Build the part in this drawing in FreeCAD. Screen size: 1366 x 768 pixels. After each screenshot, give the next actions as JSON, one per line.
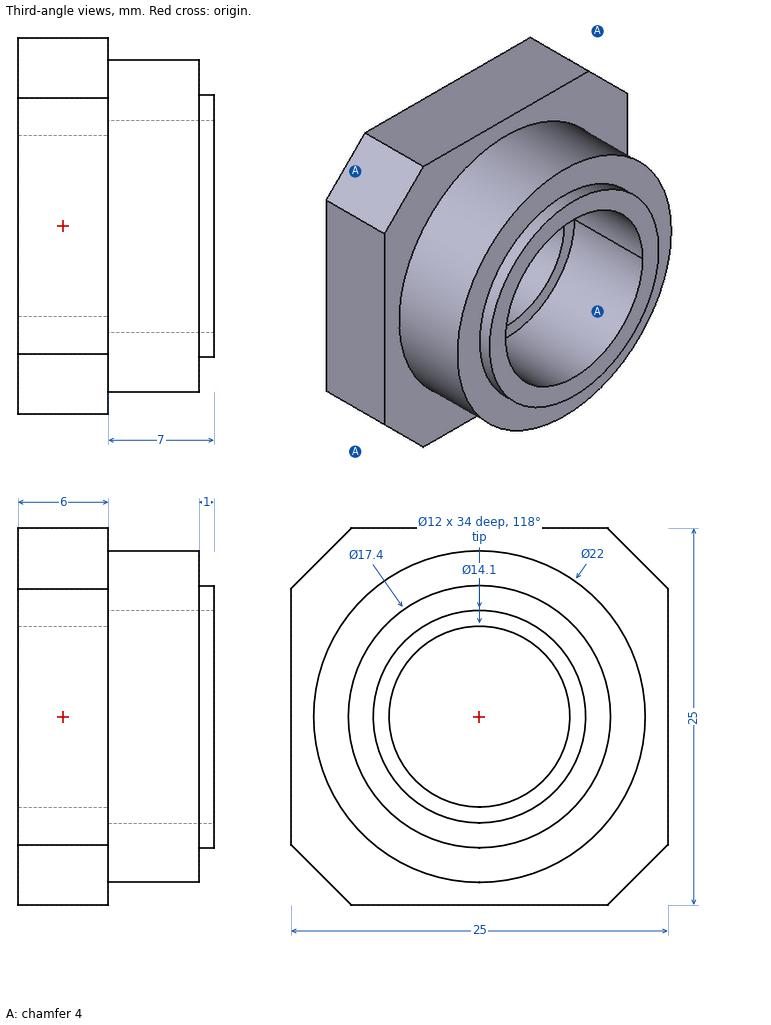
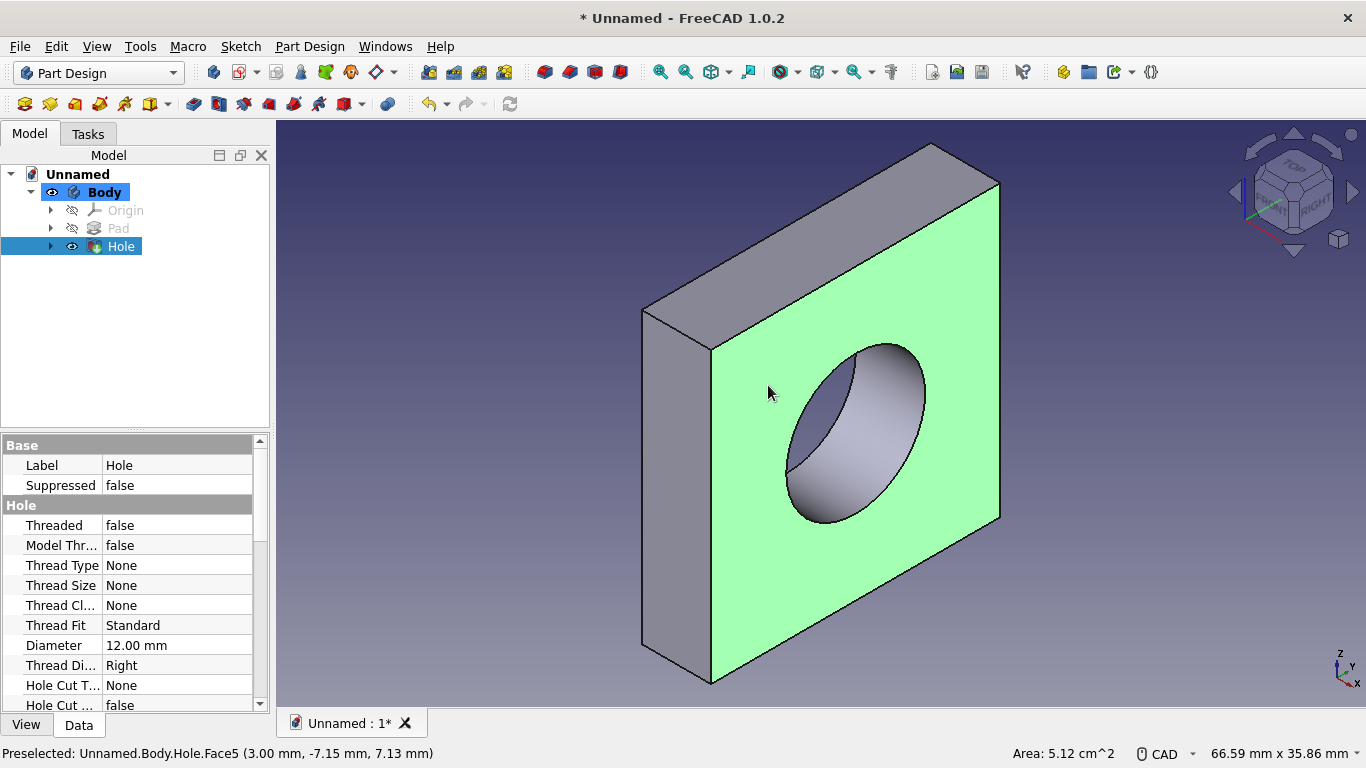
{"action": "left_click", "coordinate": [238, 72]}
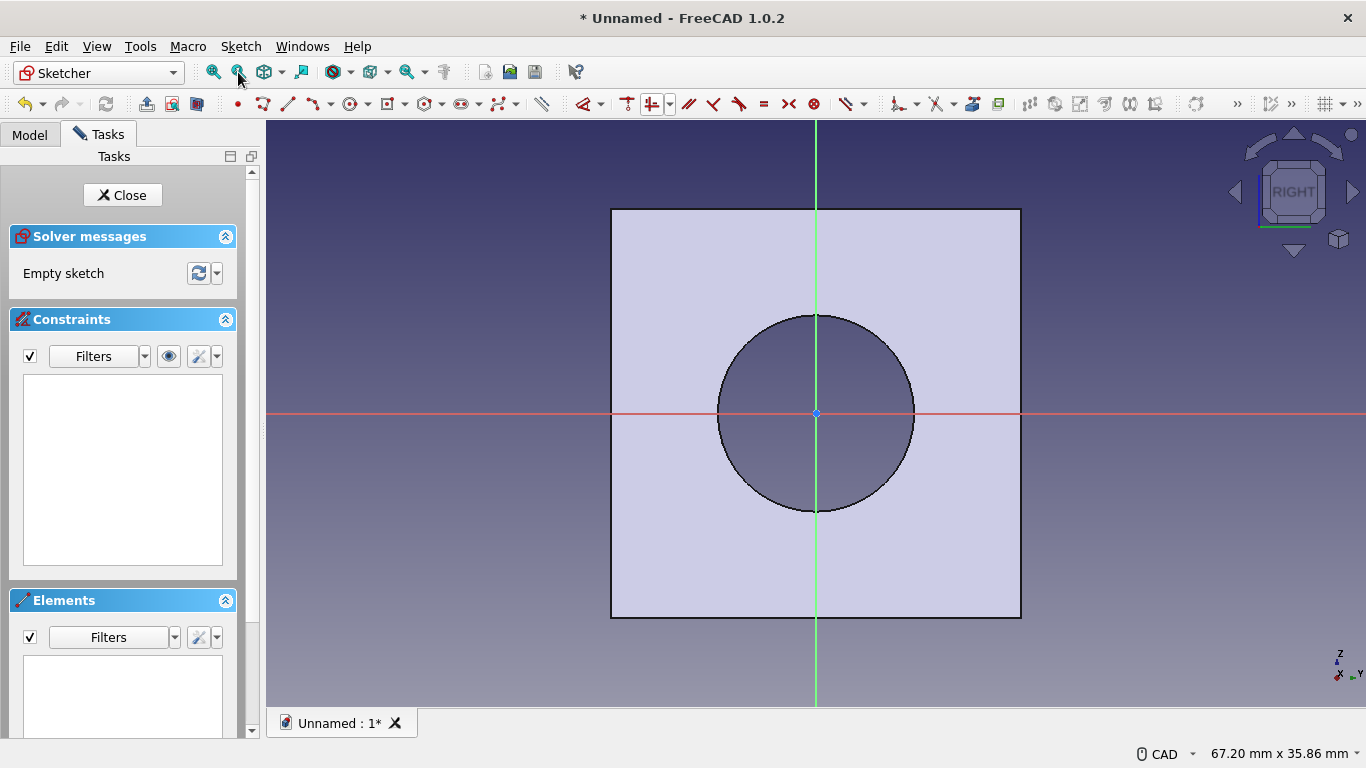
{"action": "left_click", "coordinate": [350, 104]}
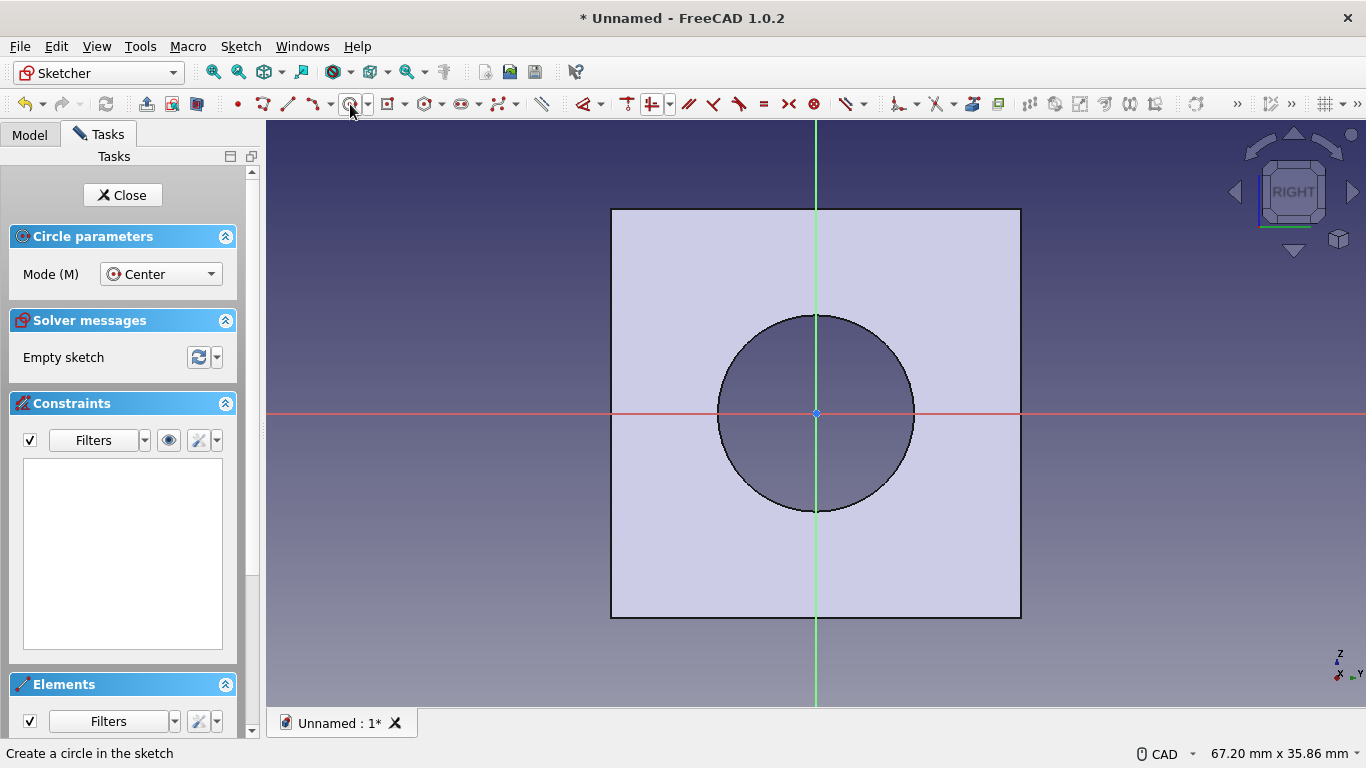
{"action": "left_click", "coordinate": [816, 414]}
{"action": "mouse_move", "coordinate": [943, 286]}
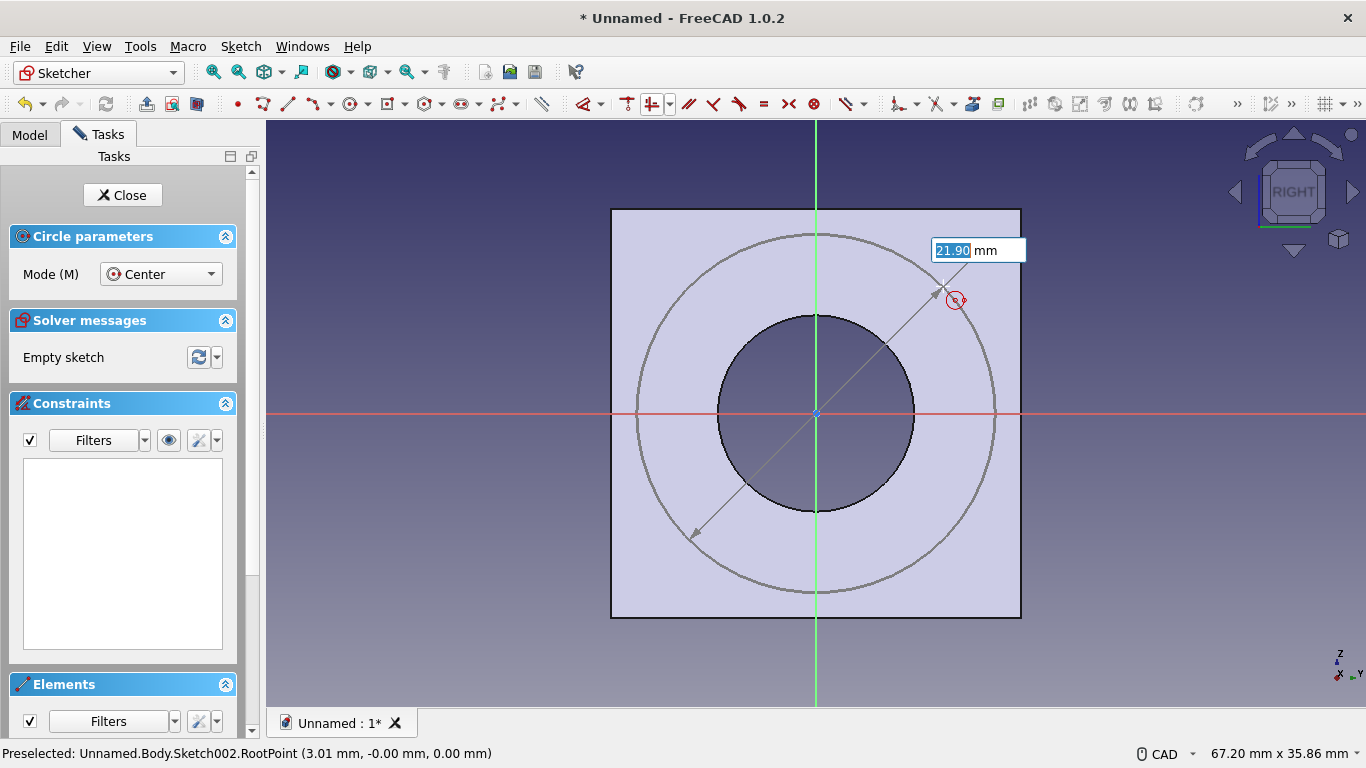
{"action": "type", "text": "22"}
{"action": "key", "text": "Return"}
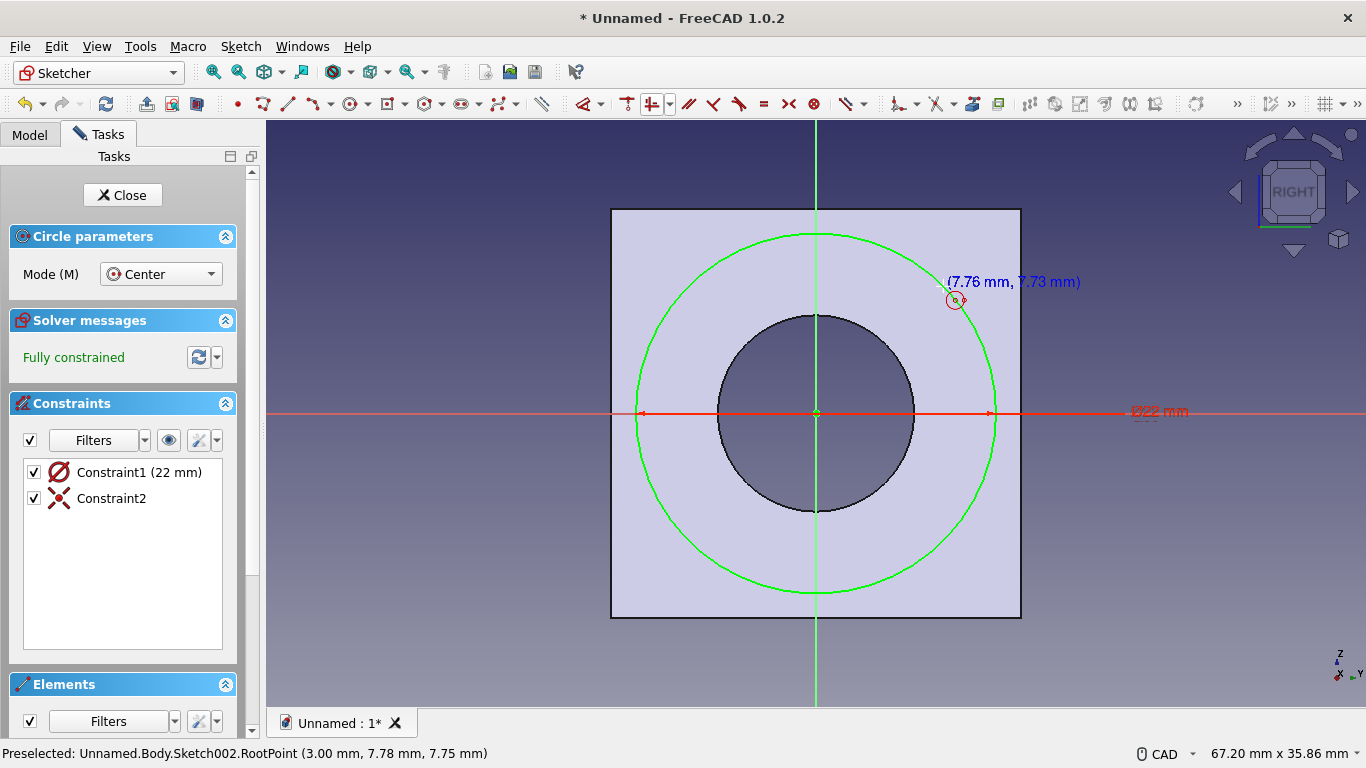
{"action": "left_click", "coordinate": [816, 414]}
{"action": "mouse_move", "coordinate": [898, 332]}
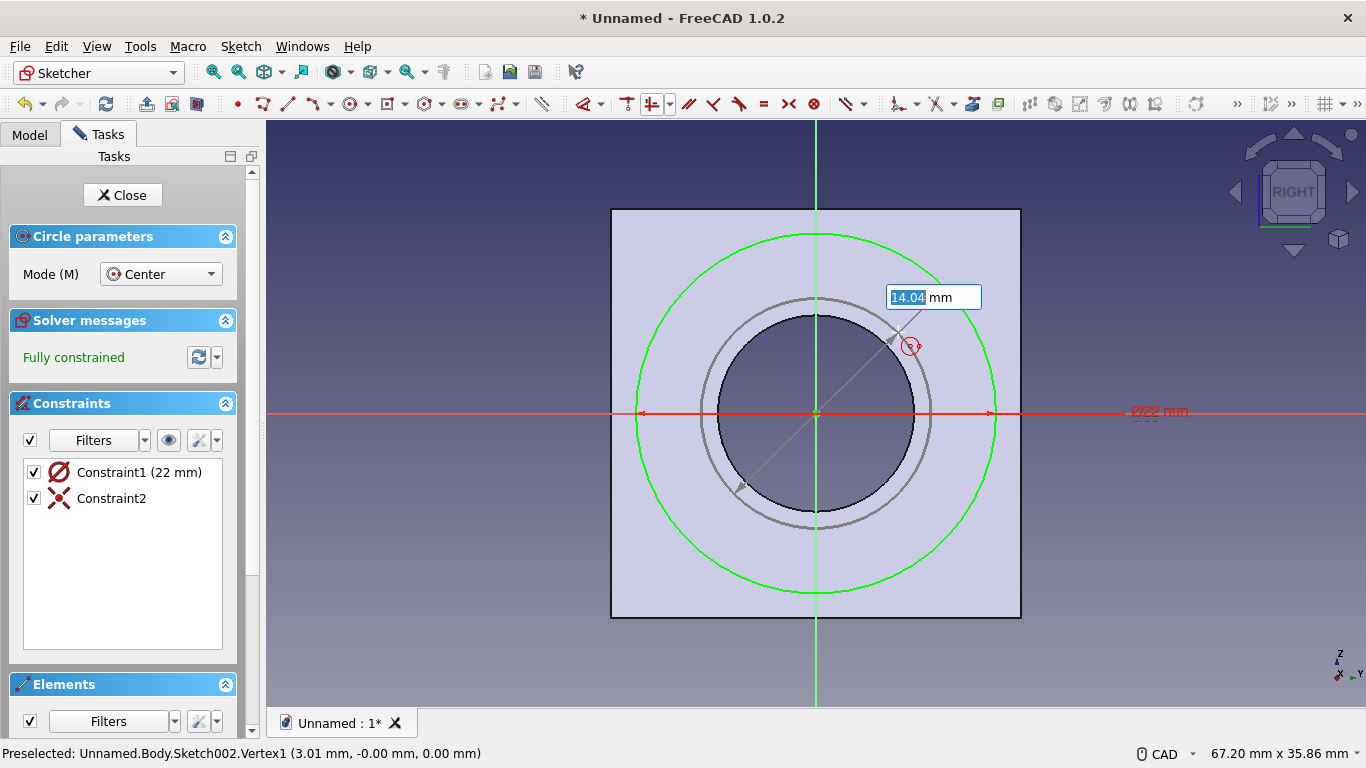
{"action": "type", "text": "14.1"}
{"action": "key", "text": "Return"}
{"action": "key", "text": "Escape"}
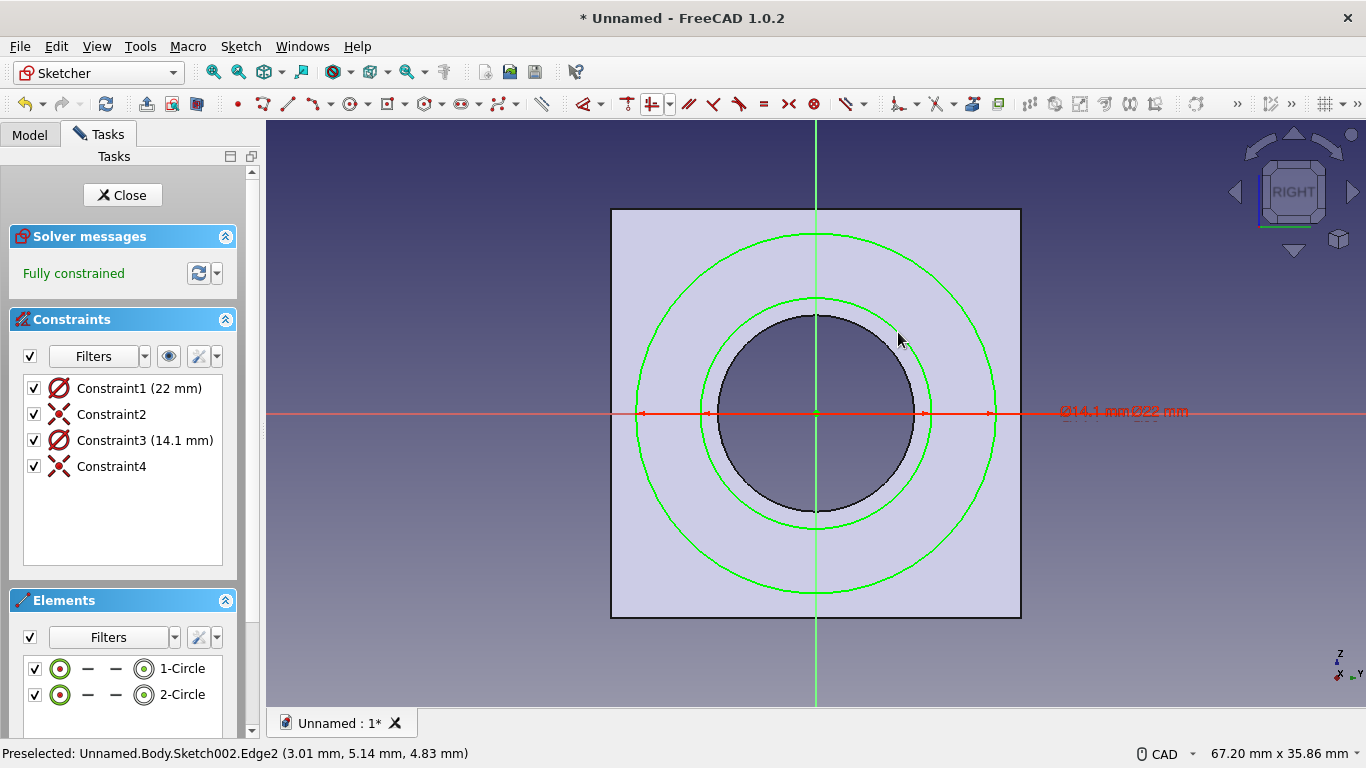
{"action": "left_click", "coordinate": [123, 195]}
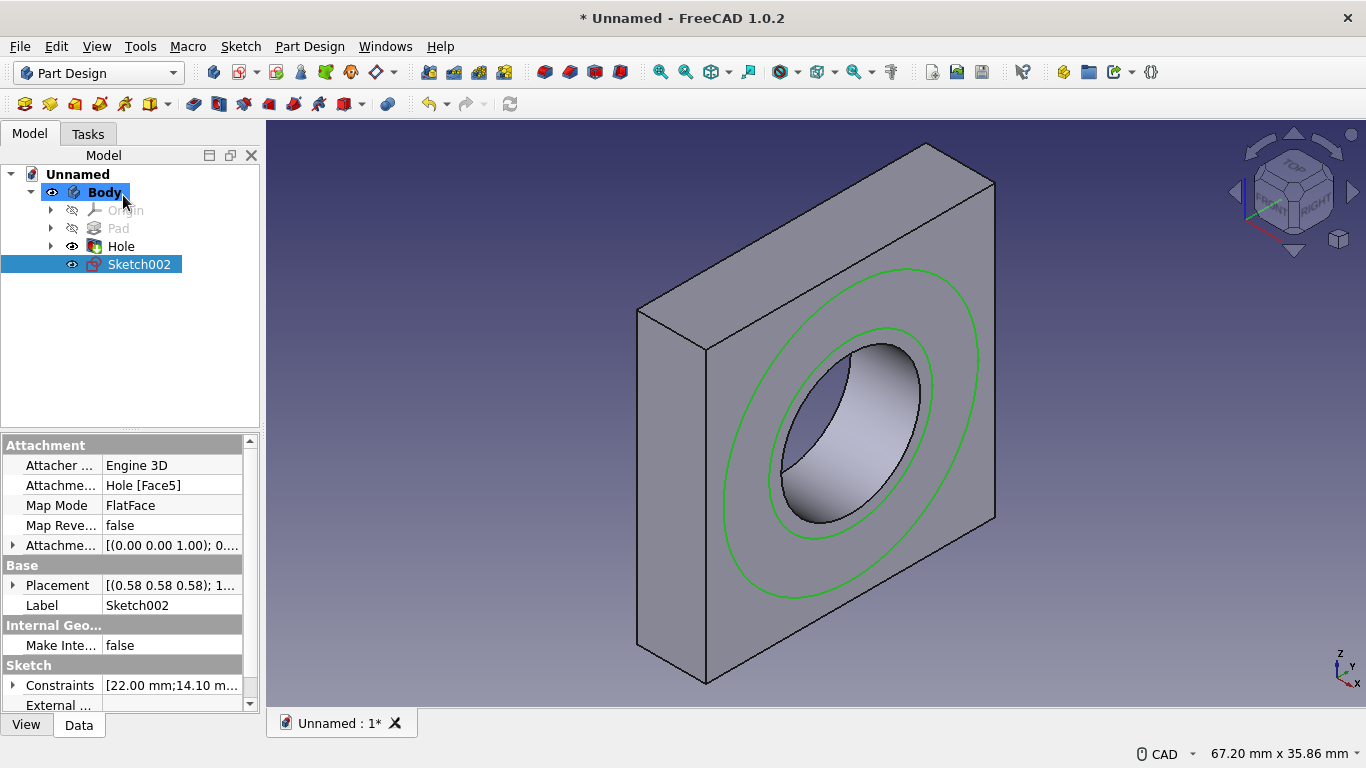
{"action": "left_click", "coordinate": [25, 104]}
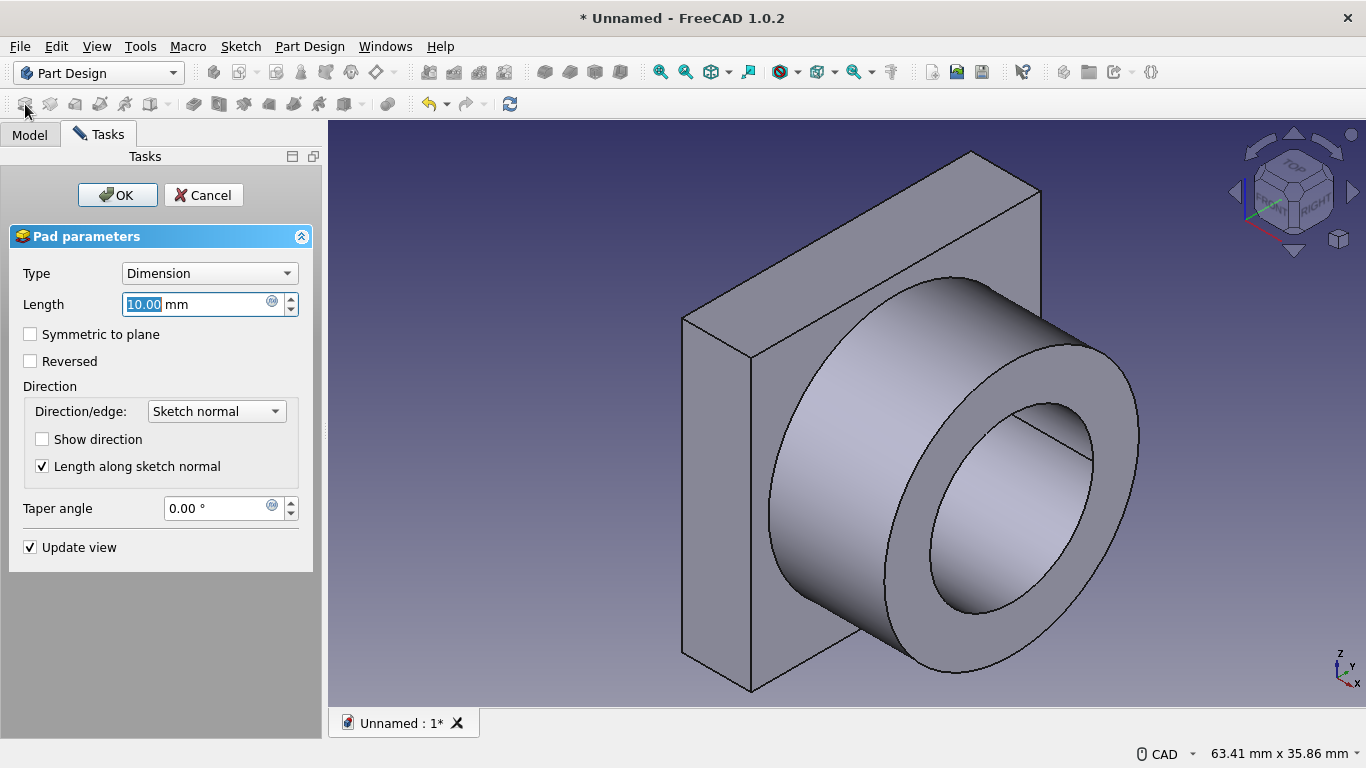
{"action": "type", "text": "7"}
{"action": "key", "text": "Tab"}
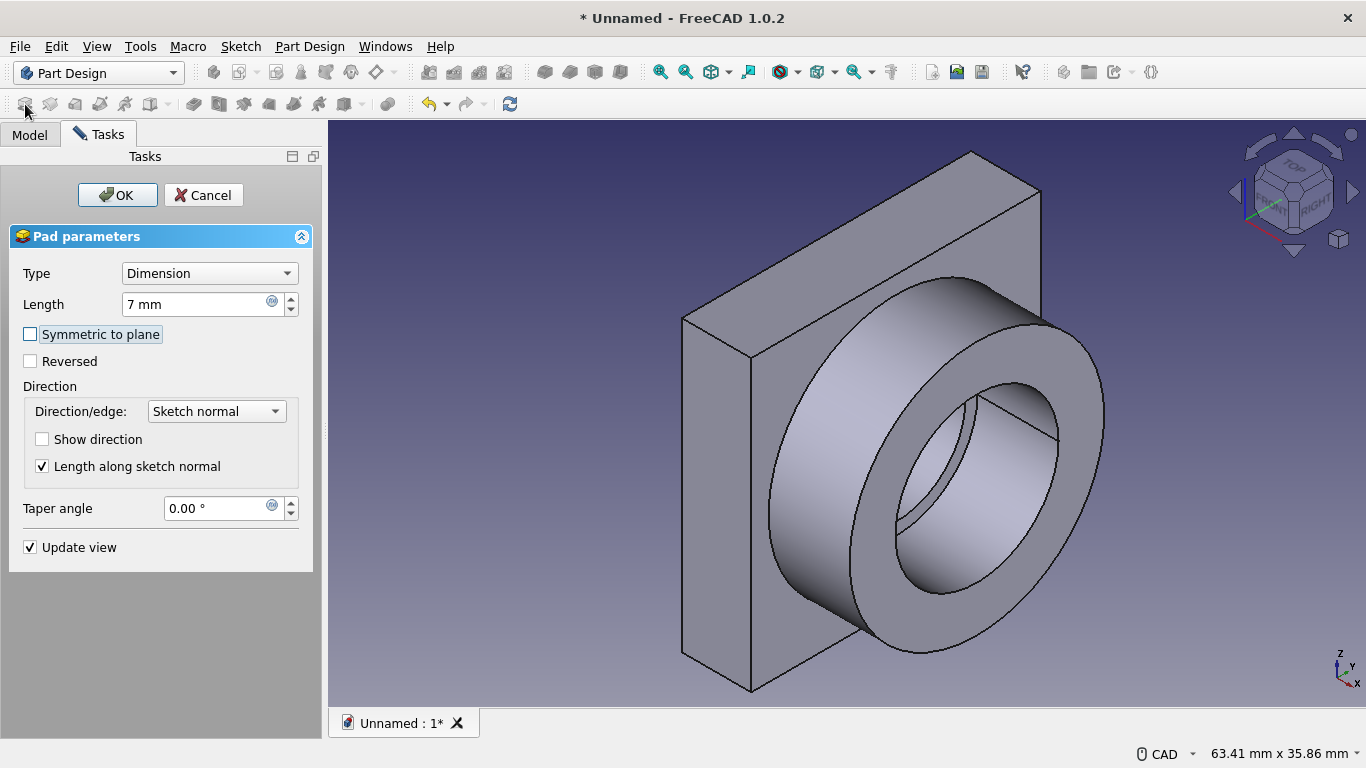
{"action": "left_click", "coordinate": [118, 195]}